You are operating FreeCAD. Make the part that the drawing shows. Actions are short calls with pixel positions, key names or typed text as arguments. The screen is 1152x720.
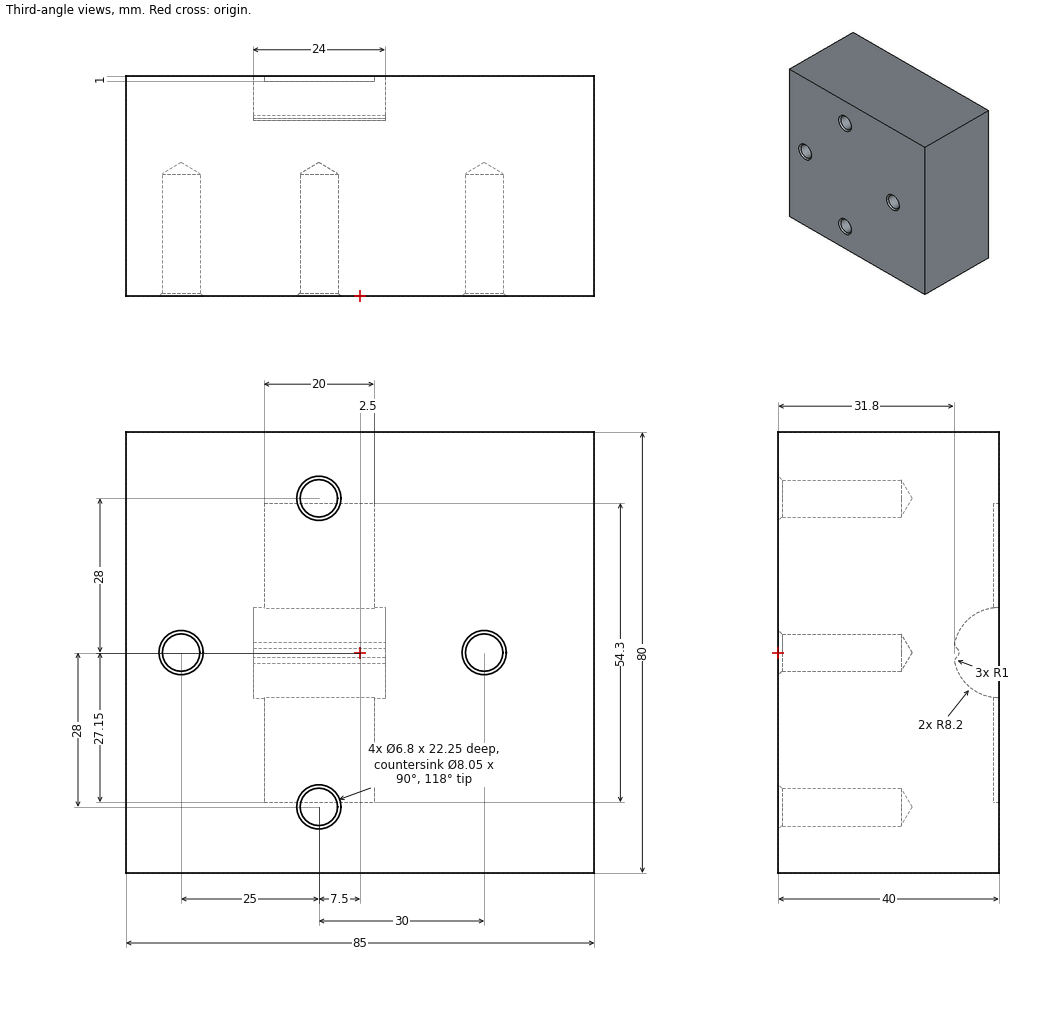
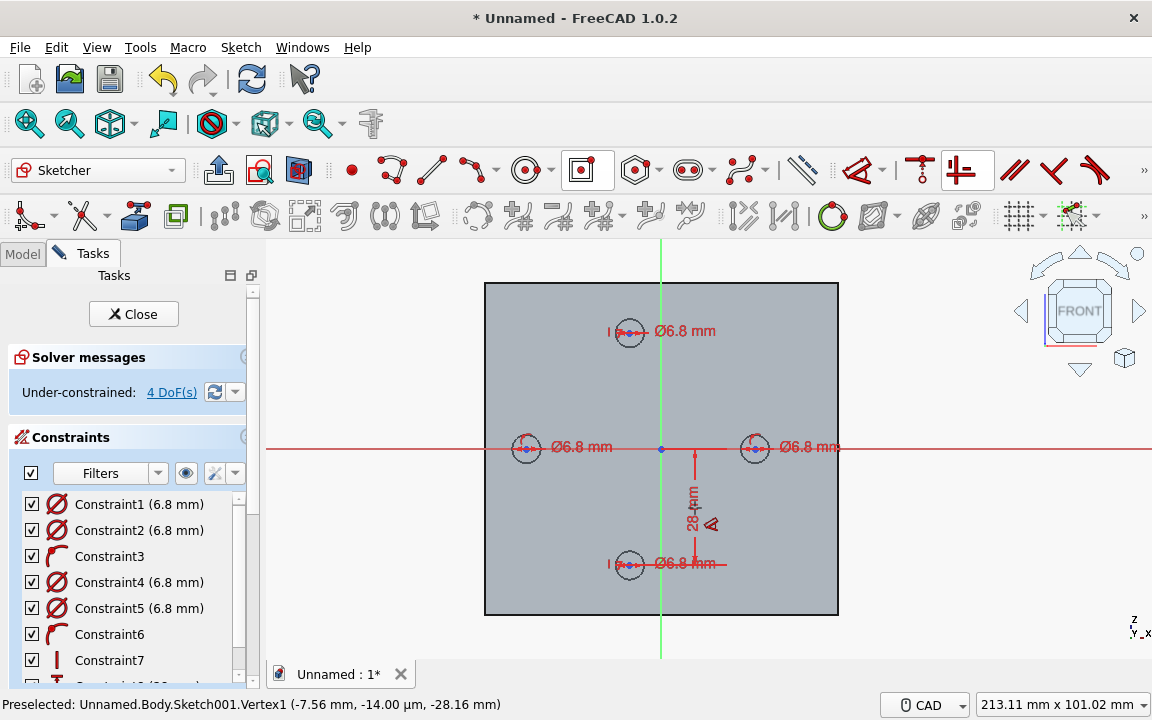
click(630, 333)
click(695, 391)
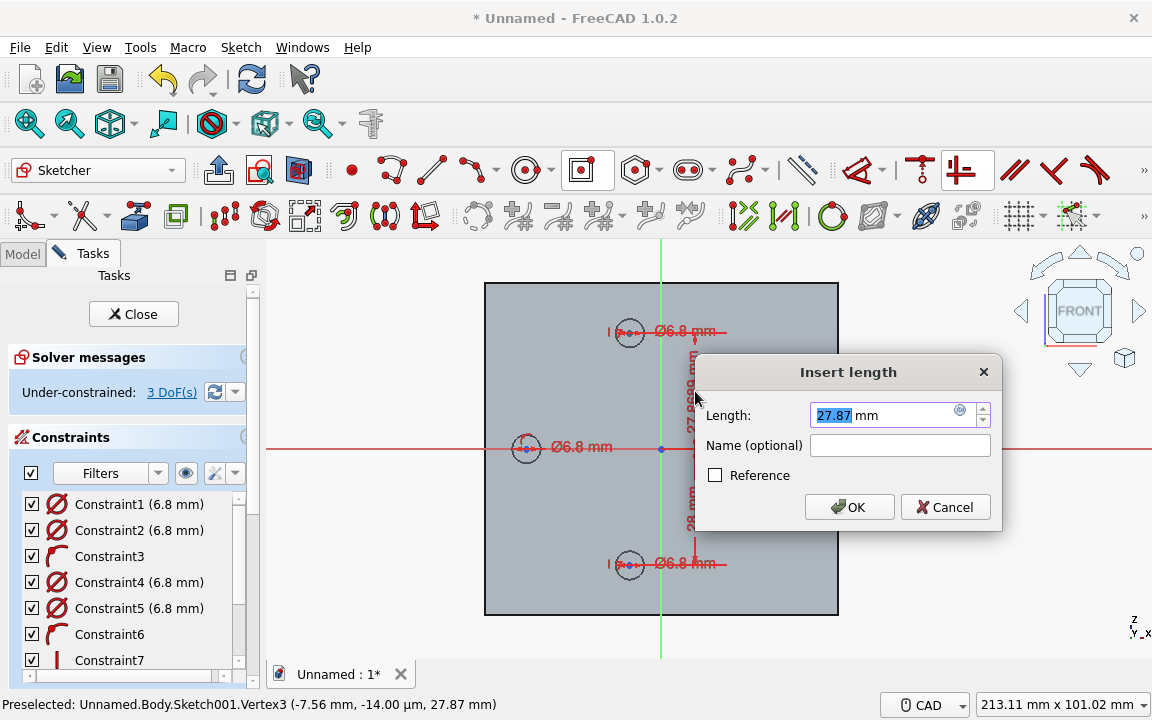
text(28)
key(Return)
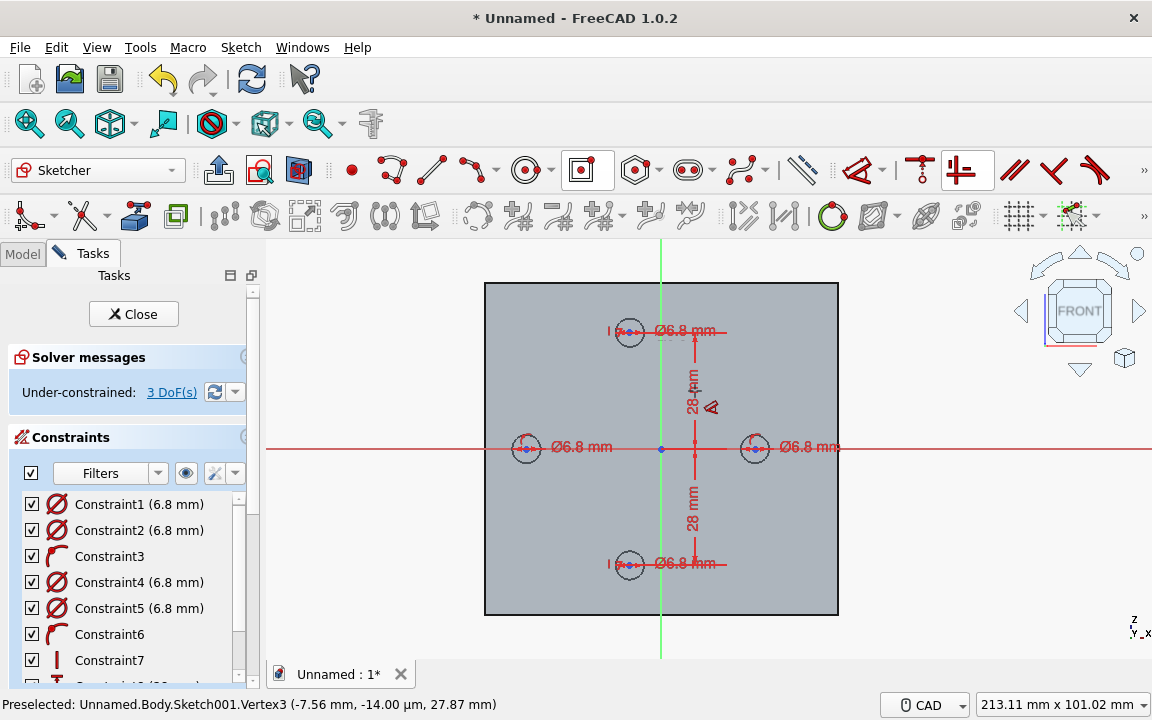
scroll(630, 565, up, 2)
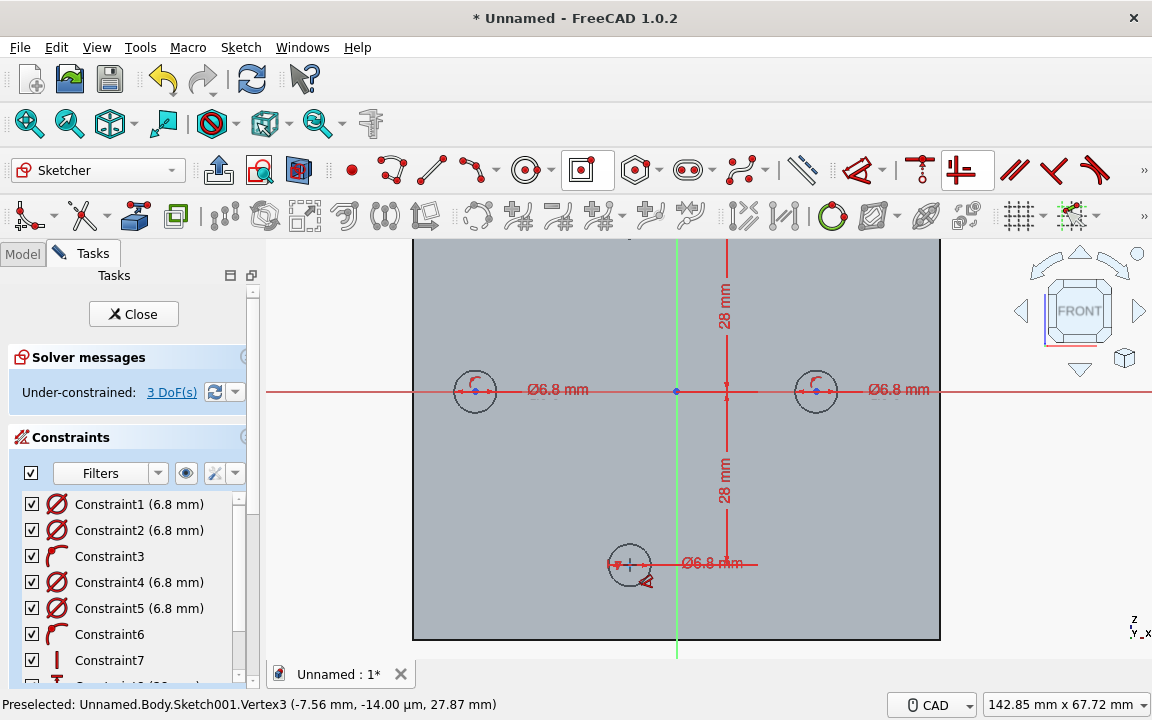
click(630, 565)
click(653, 599)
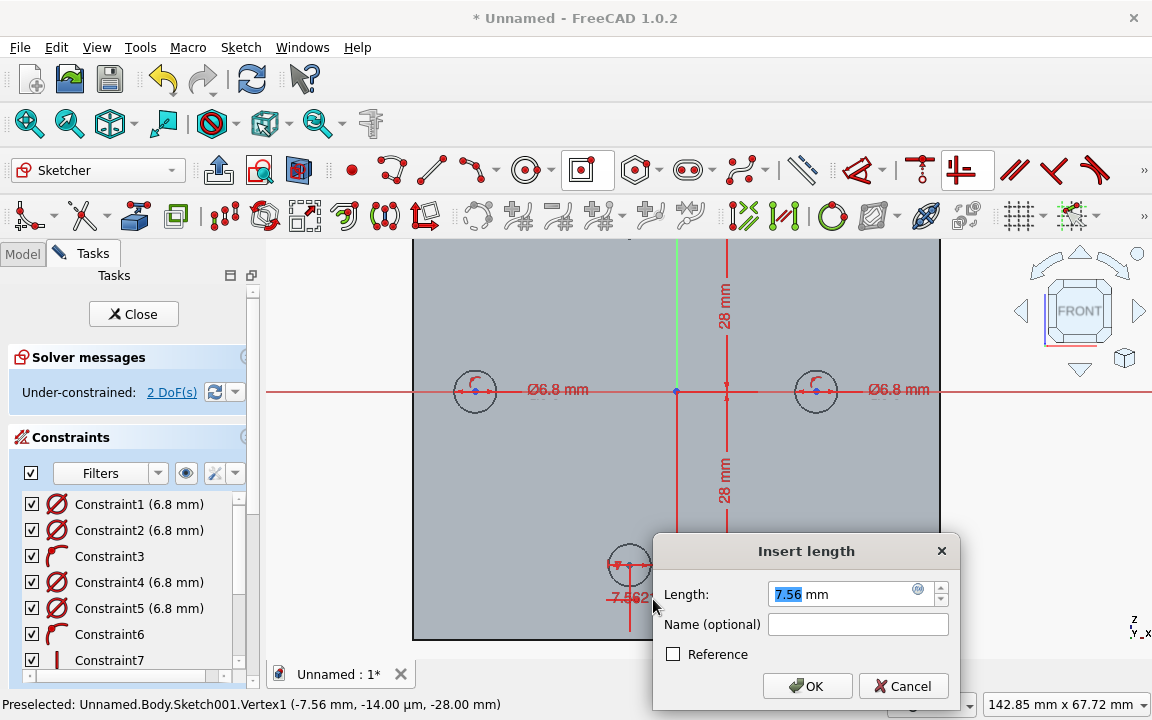
text(7.5)
key(Return)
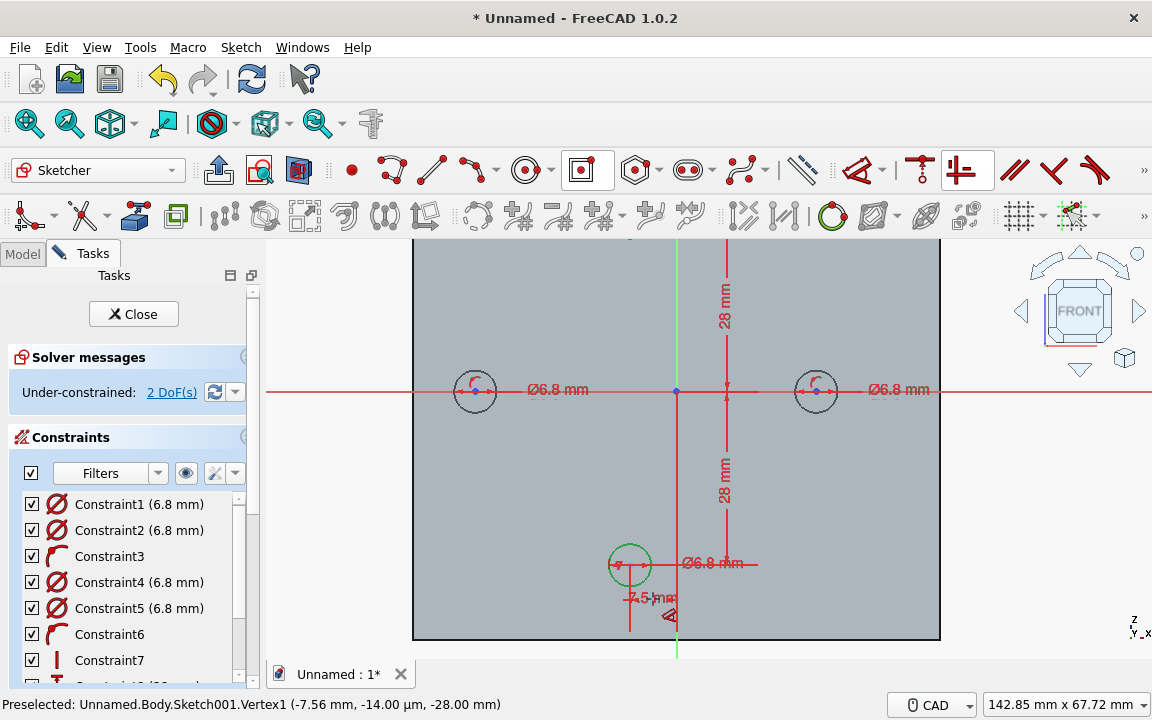
click(630, 565)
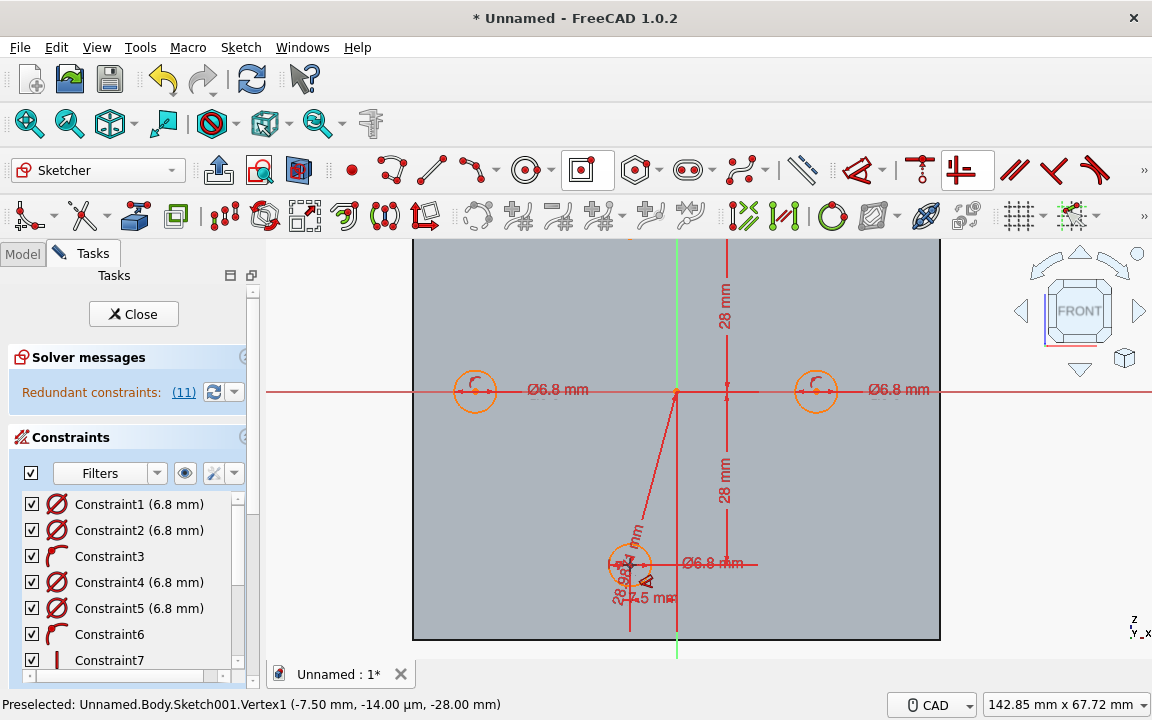
click(816, 392)
click(723, 599)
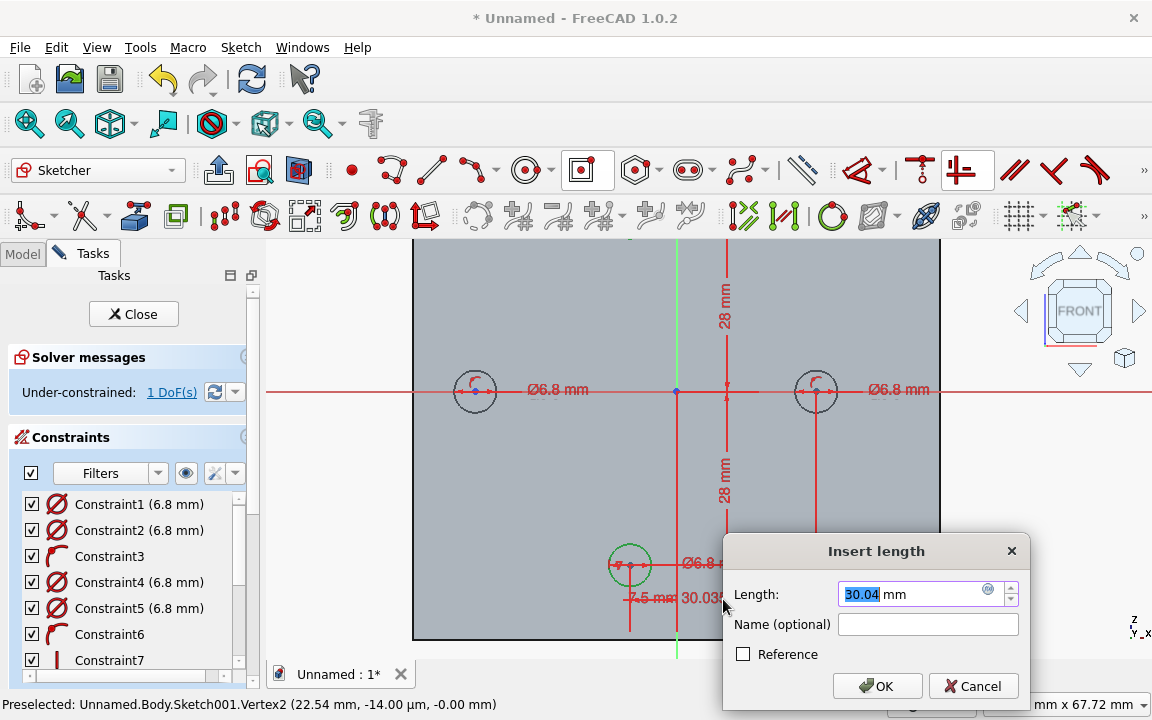
text(30)
key(Return)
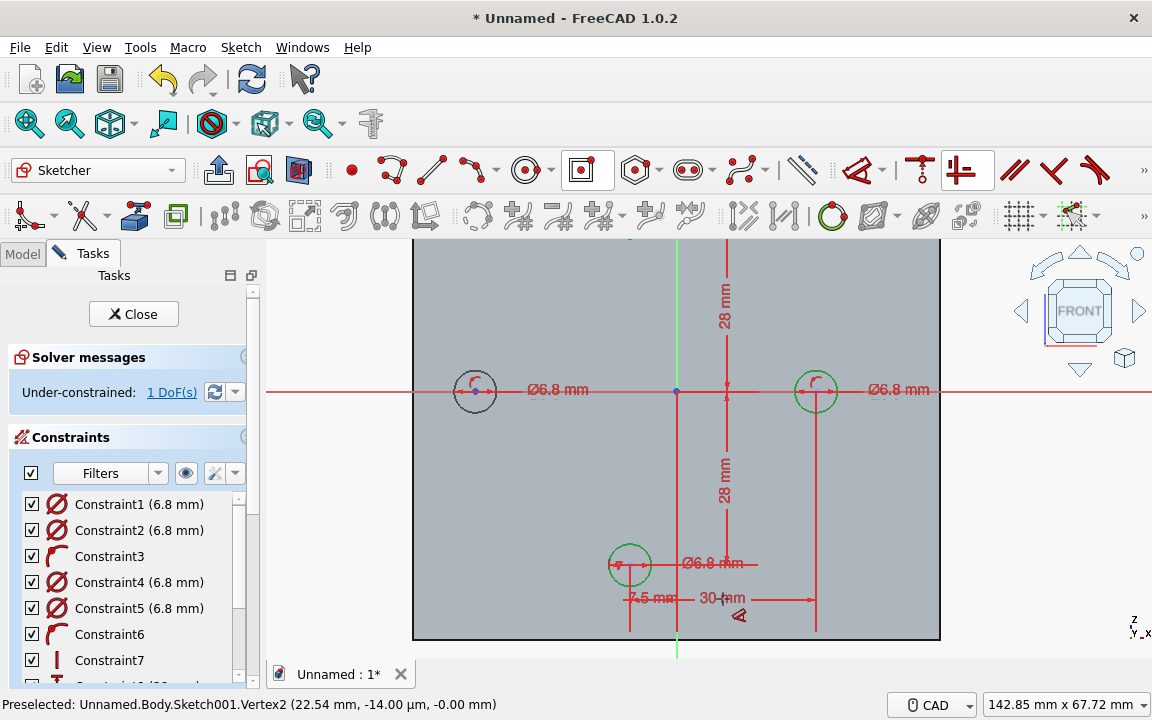
click(630, 565)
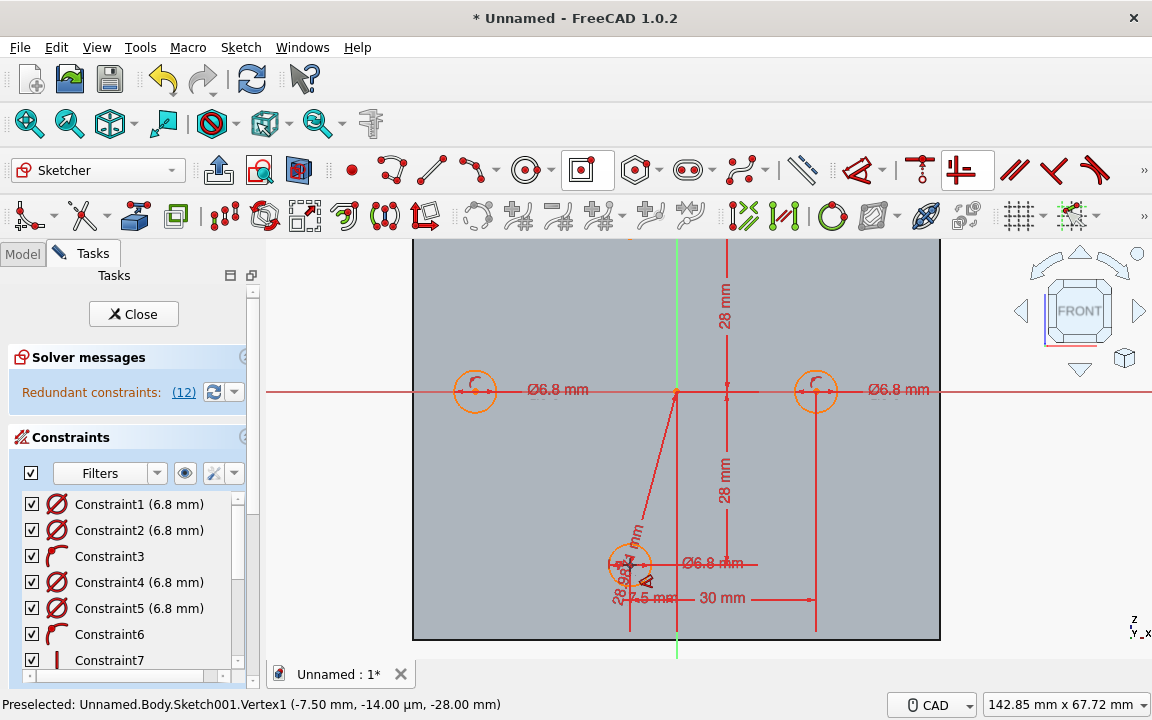
click(475, 392)
click(553, 599)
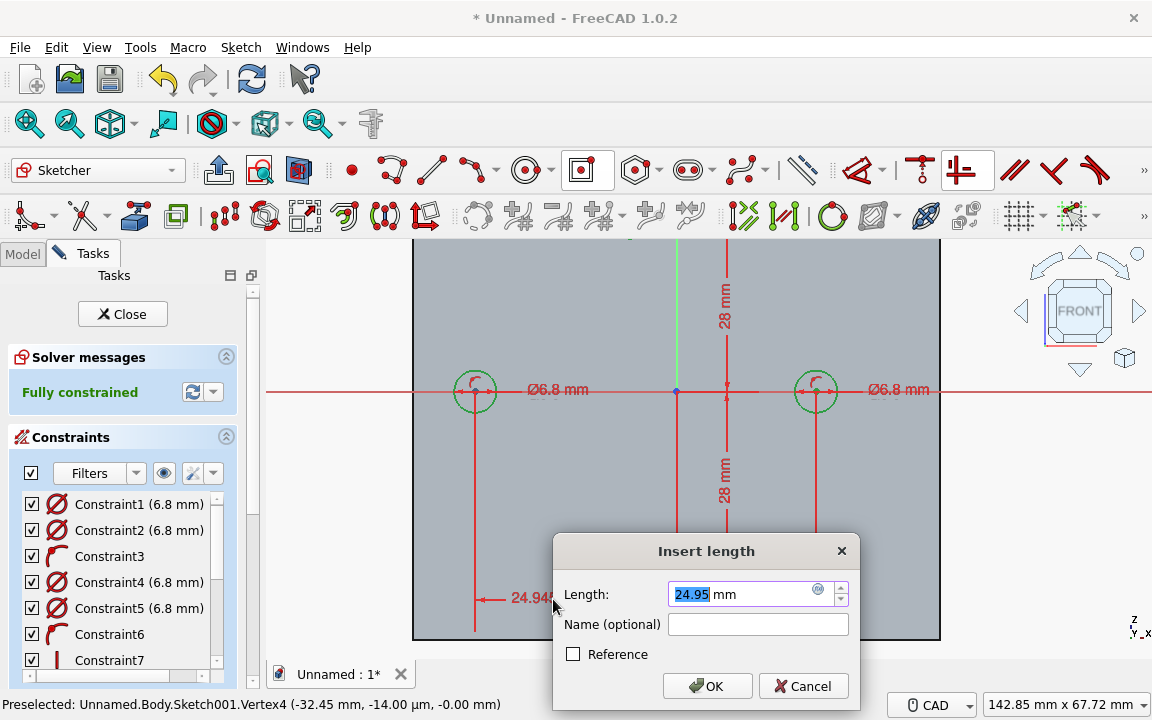
text(25)
key(Return)
key(Escape)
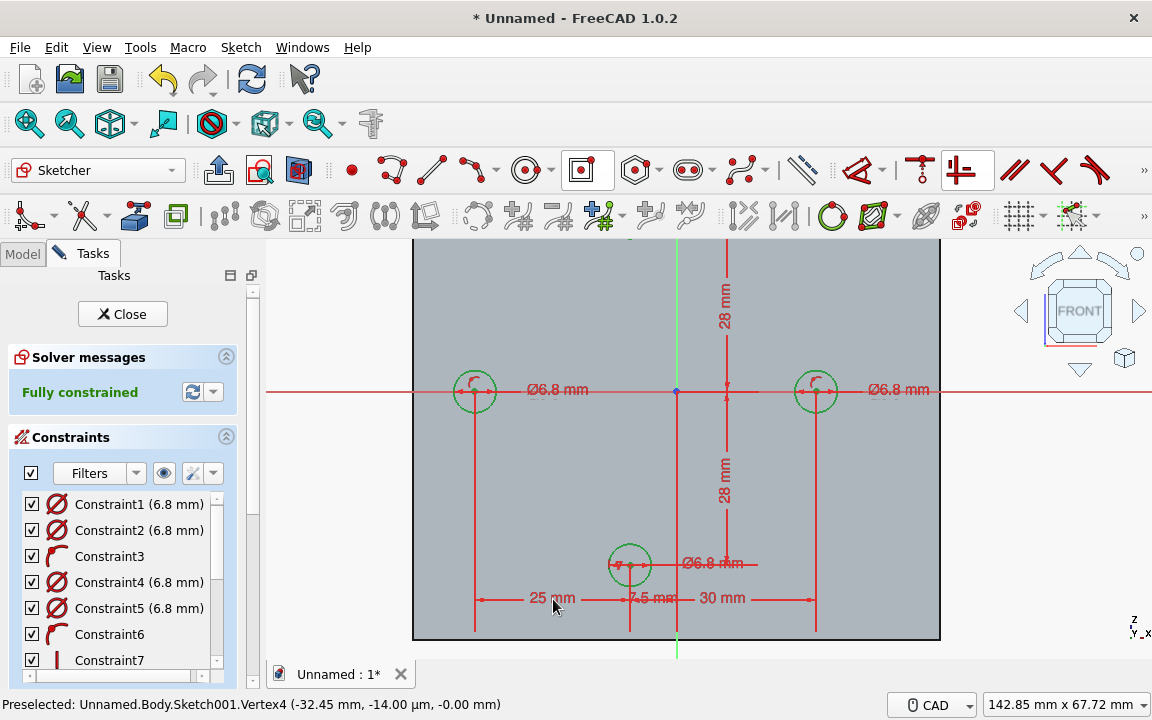
click(123, 314)